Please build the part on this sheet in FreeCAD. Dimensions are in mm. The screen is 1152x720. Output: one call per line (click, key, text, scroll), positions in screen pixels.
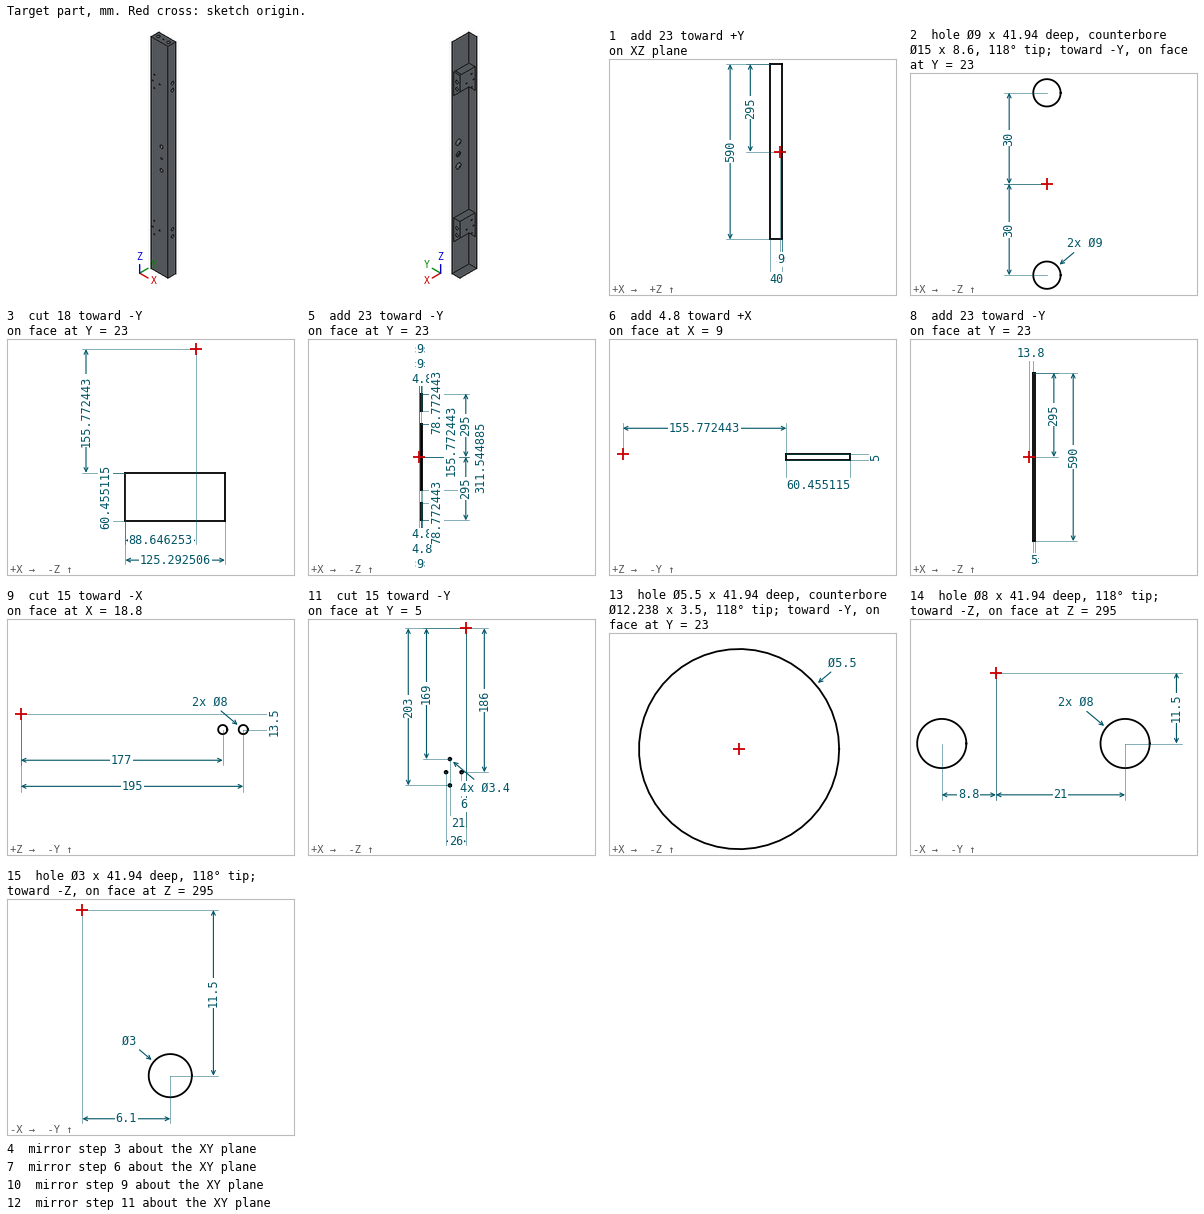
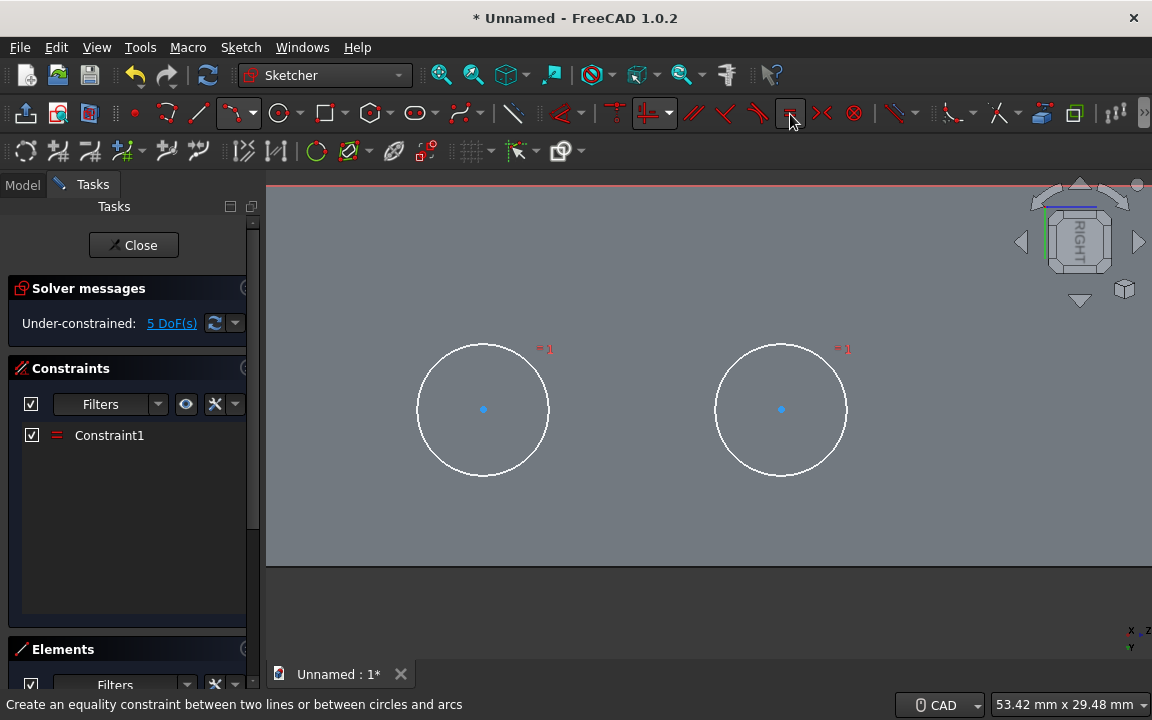
click(781, 410)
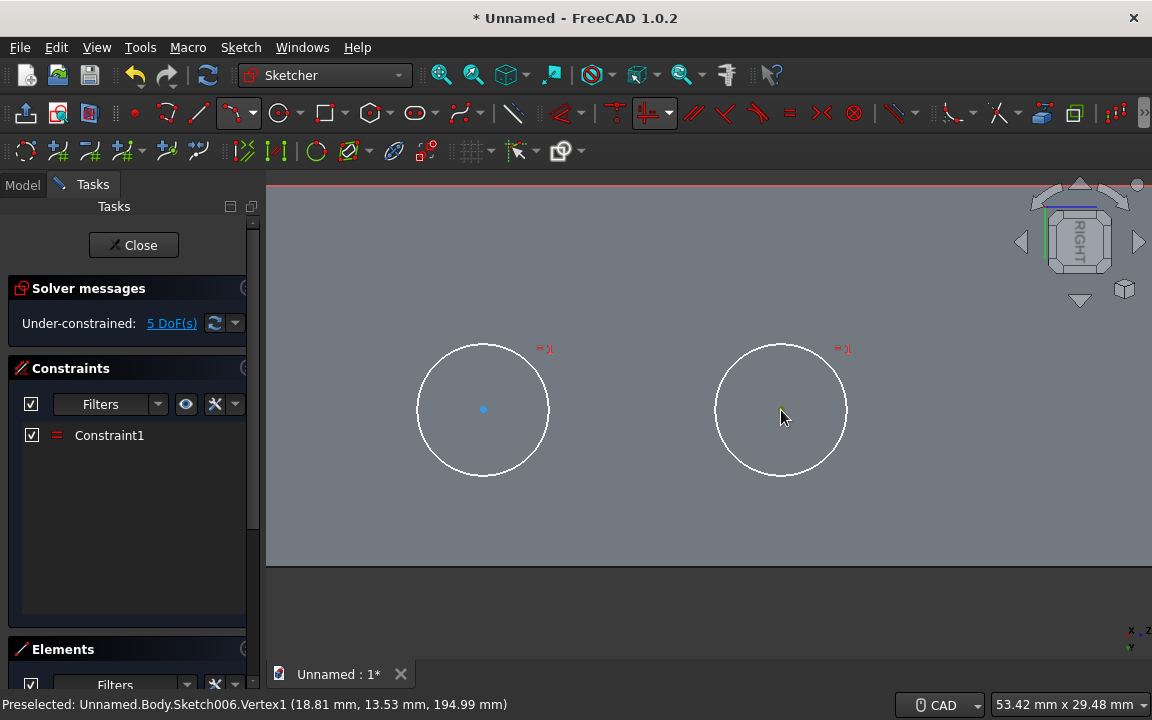
click(483, 410)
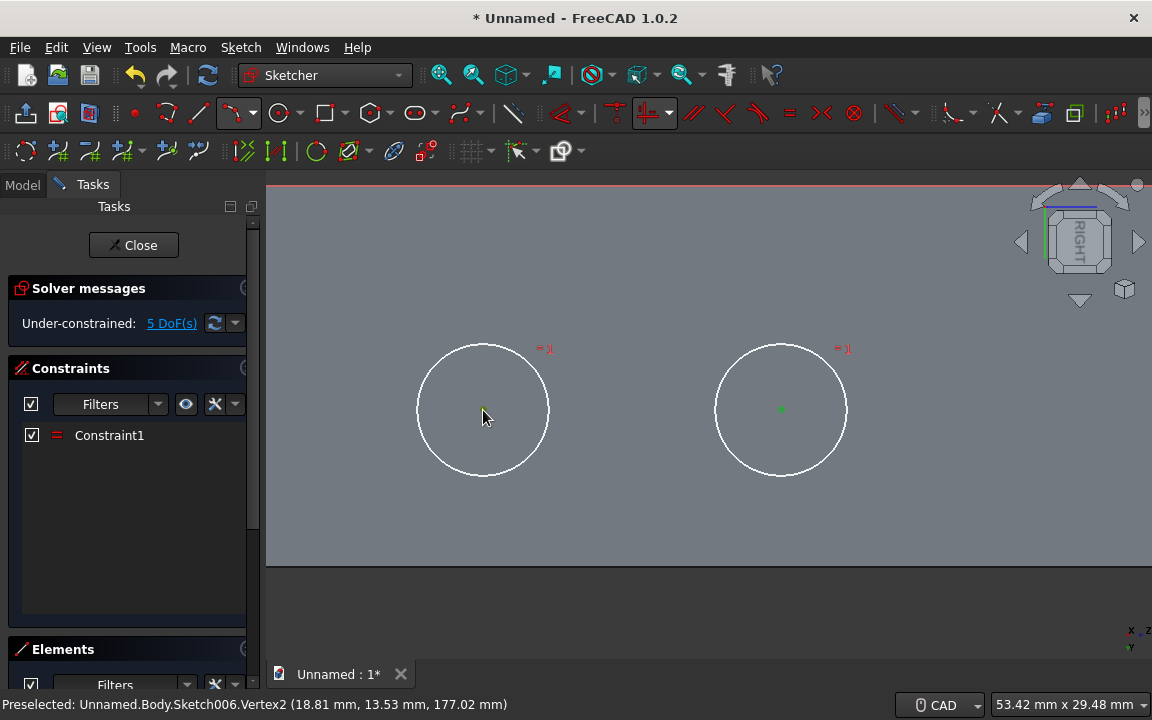
click(672, 114)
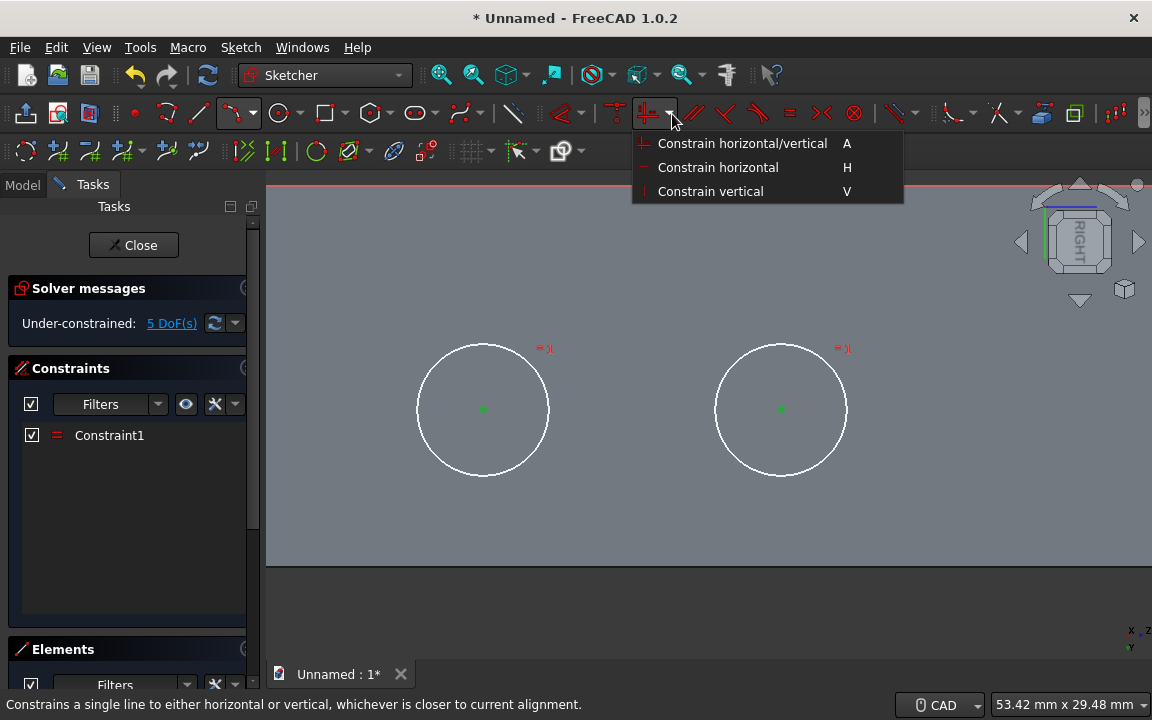
click(768, 167)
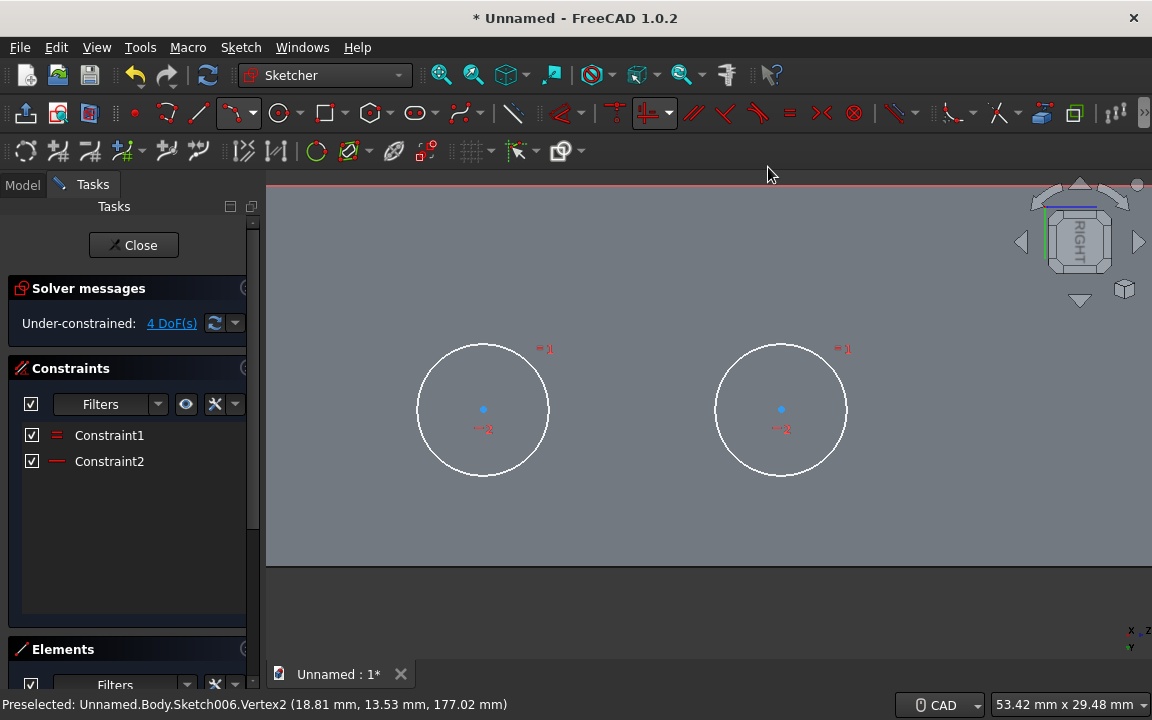
click(560, 114)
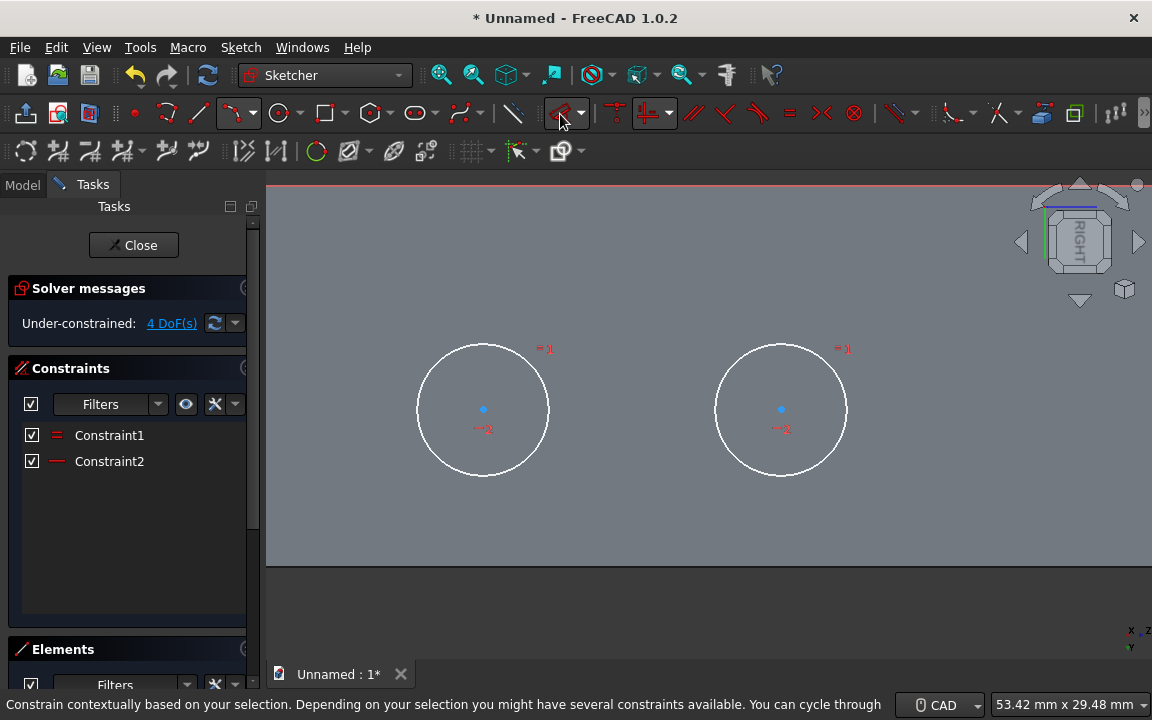
click(827, 363)
click(849, 340)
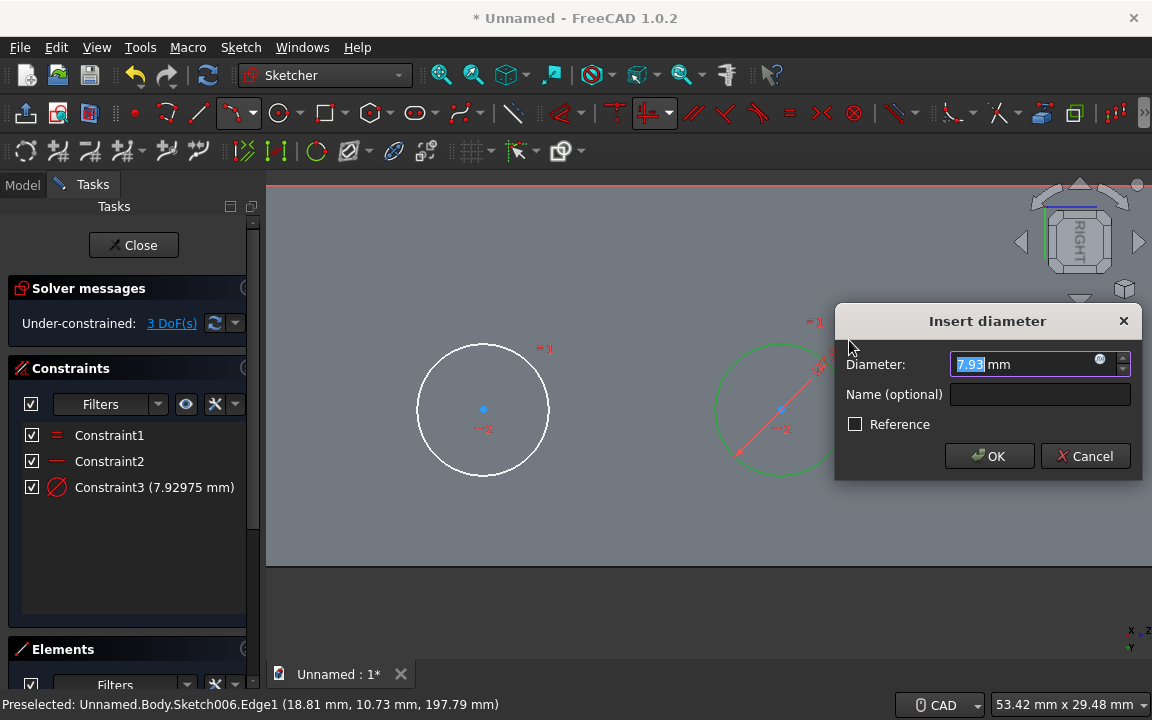
text(8)
key(Return)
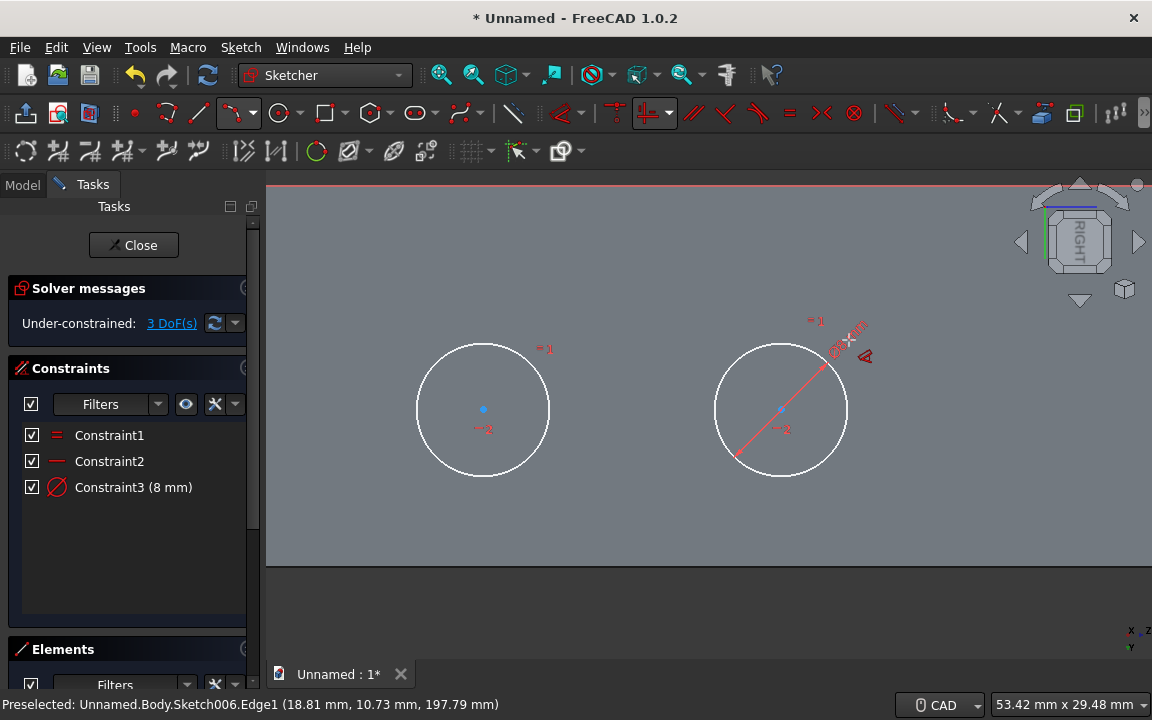
click(781, 410)
click(650, 444)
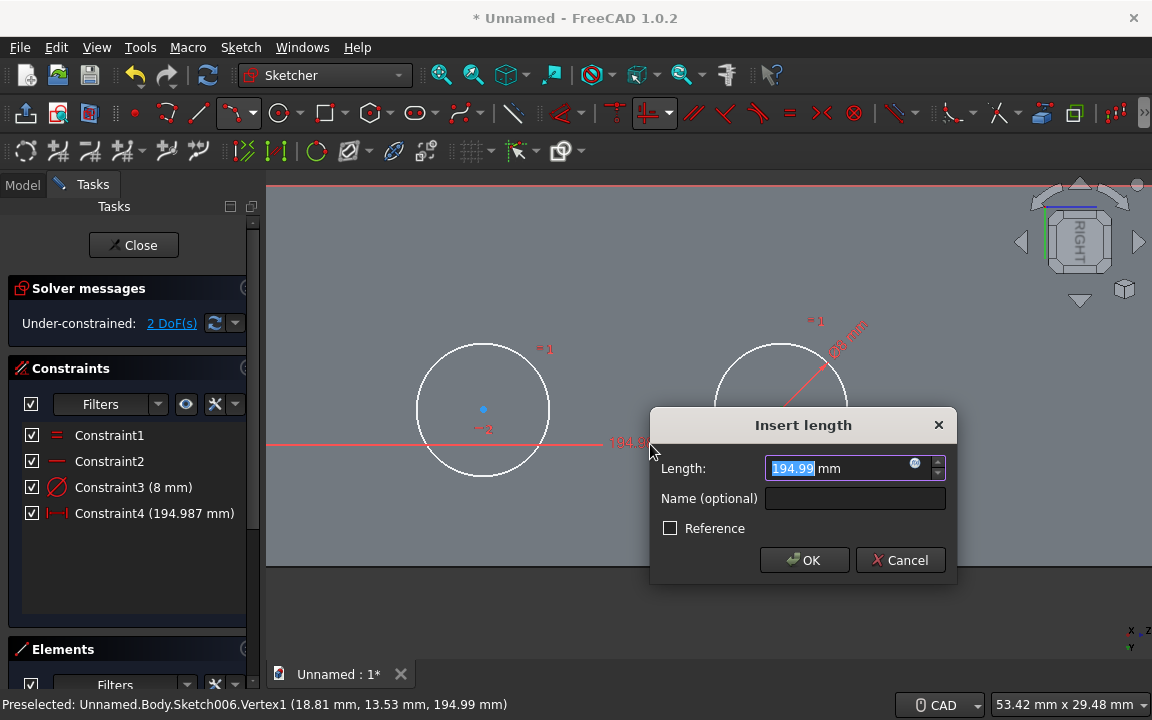
text(195)
key(Return)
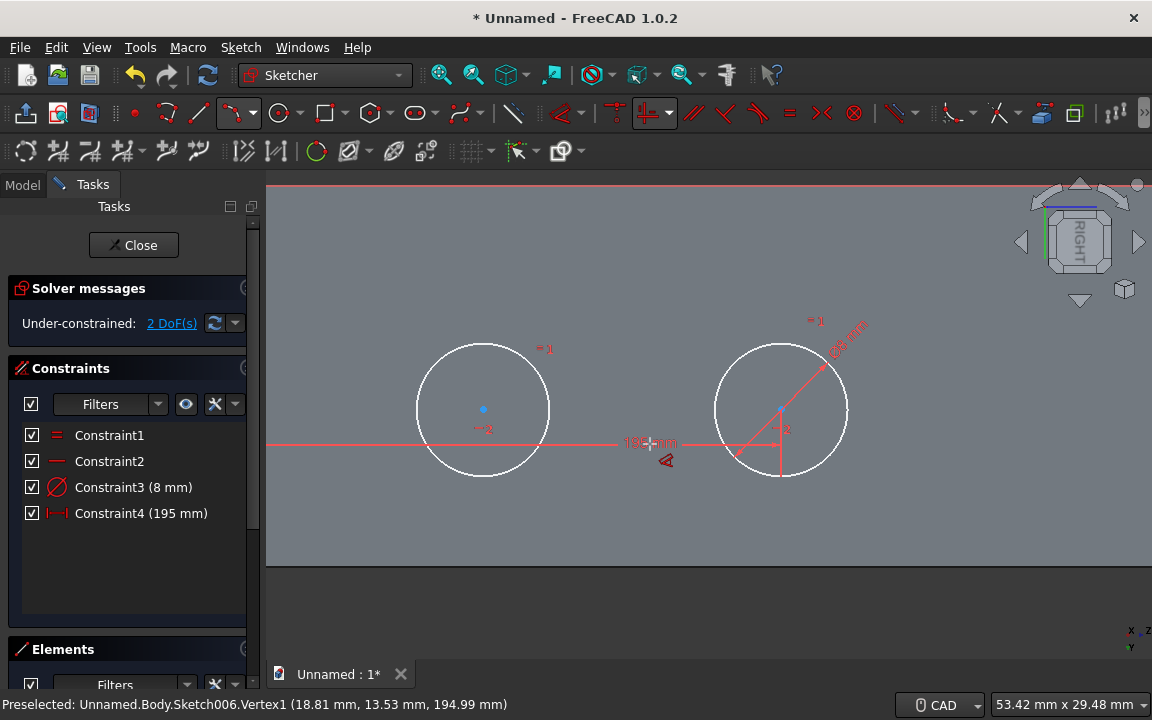
click(483, 410)
click(388, 444)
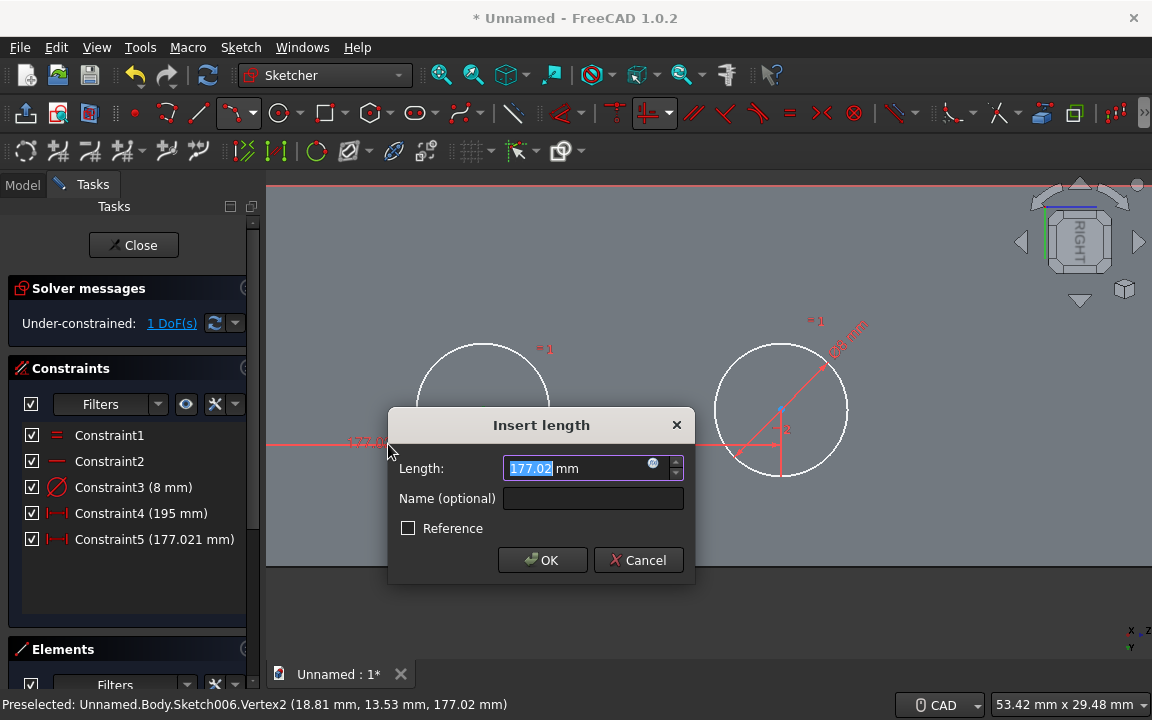
text(177)
key(Return)